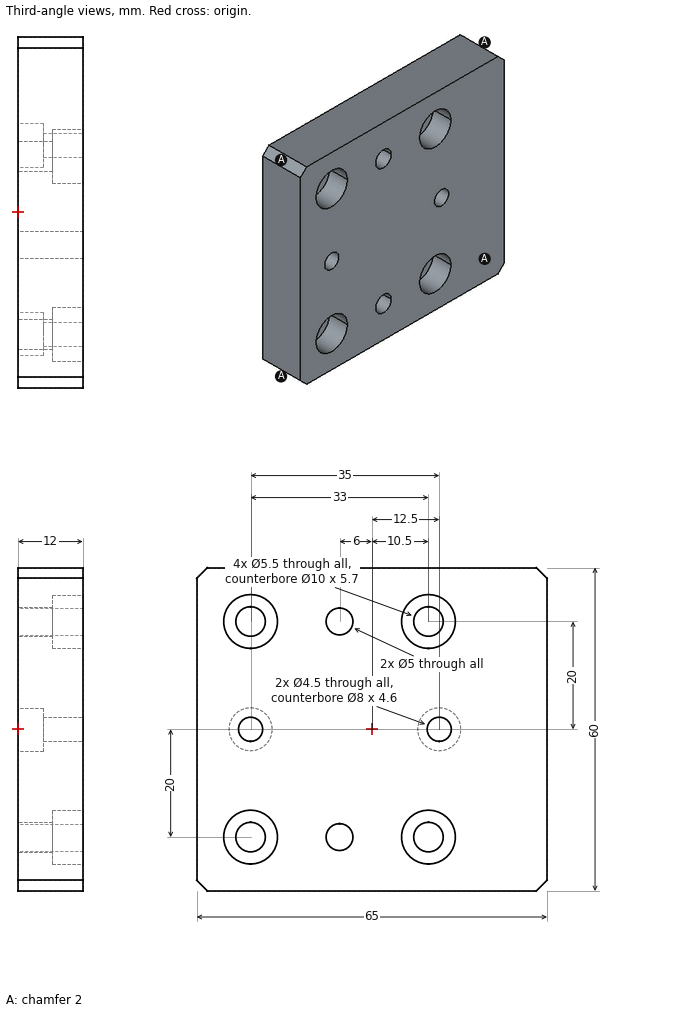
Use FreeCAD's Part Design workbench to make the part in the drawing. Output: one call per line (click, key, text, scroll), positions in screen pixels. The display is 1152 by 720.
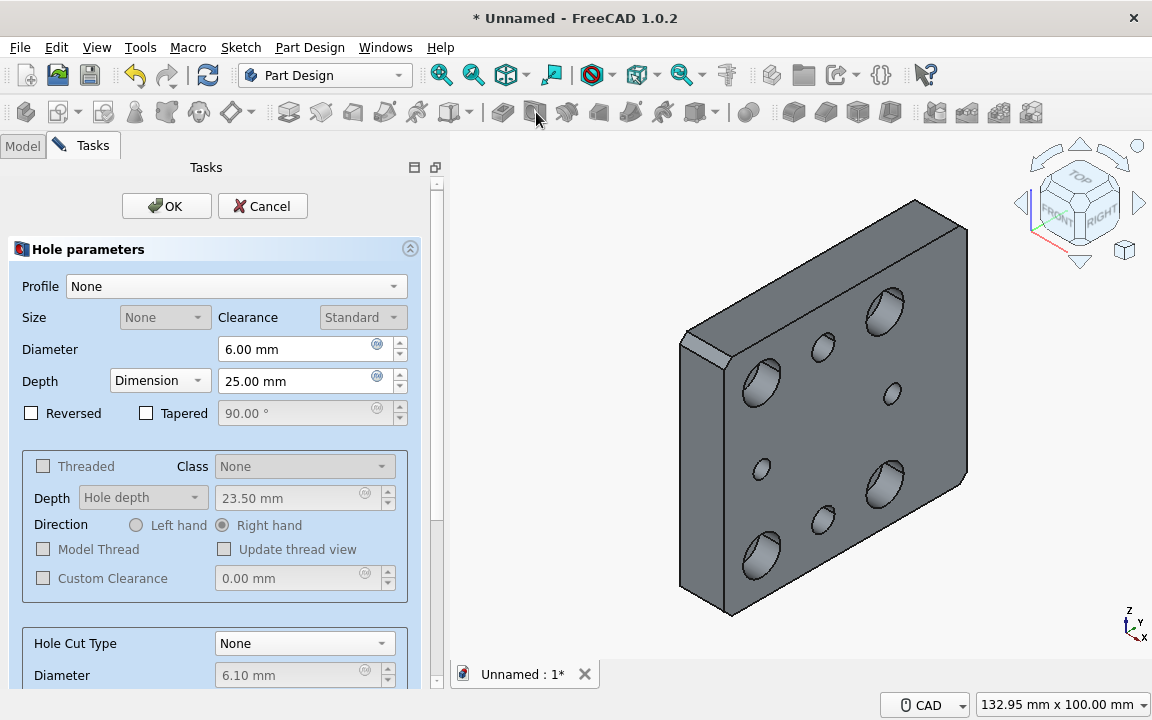
triple_click(305, 349)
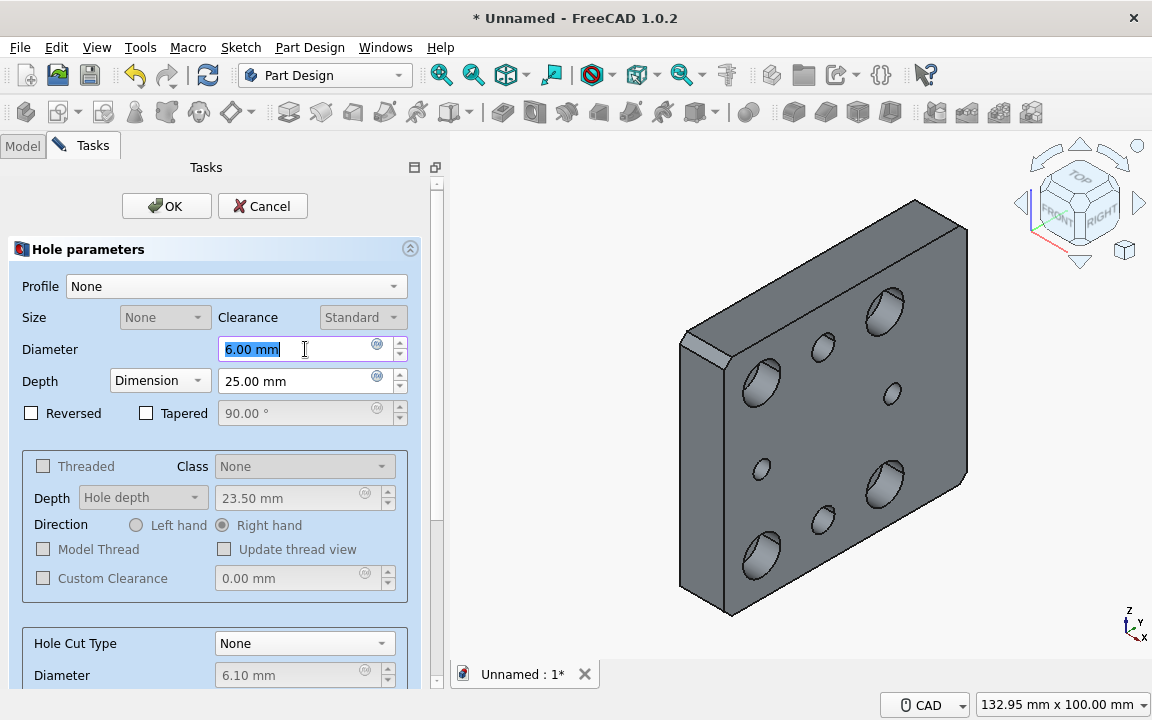
text(5)
key(Tab)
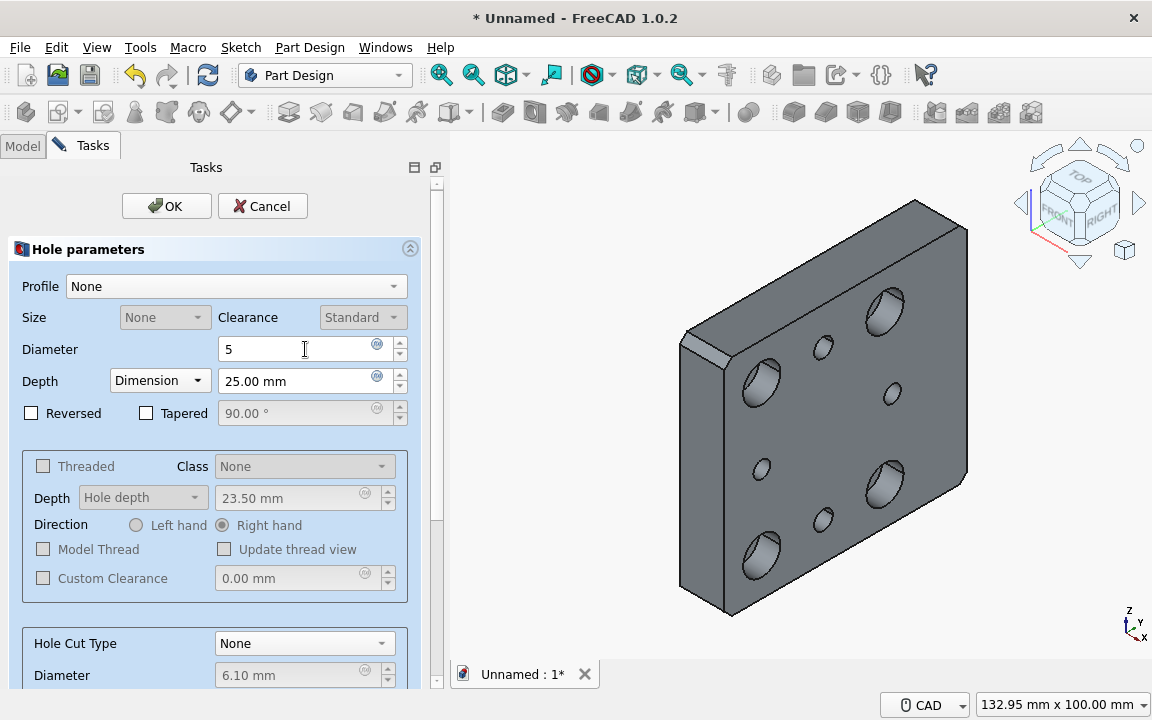
click(161, 380)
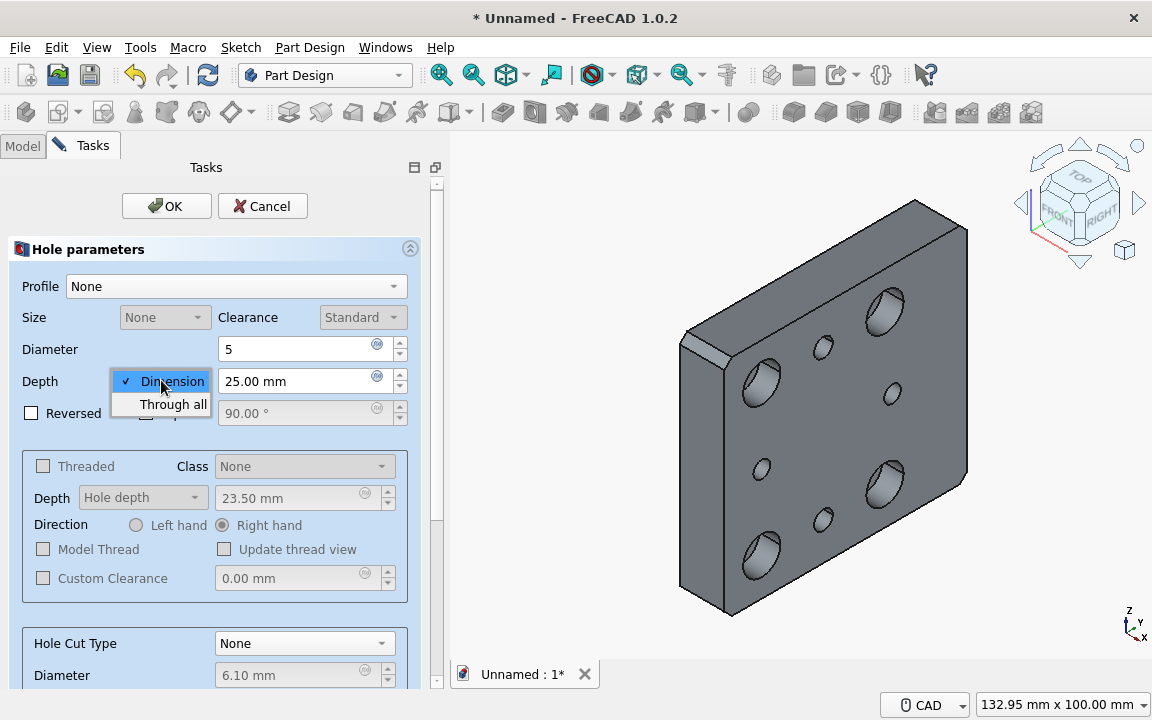
click(160, 404)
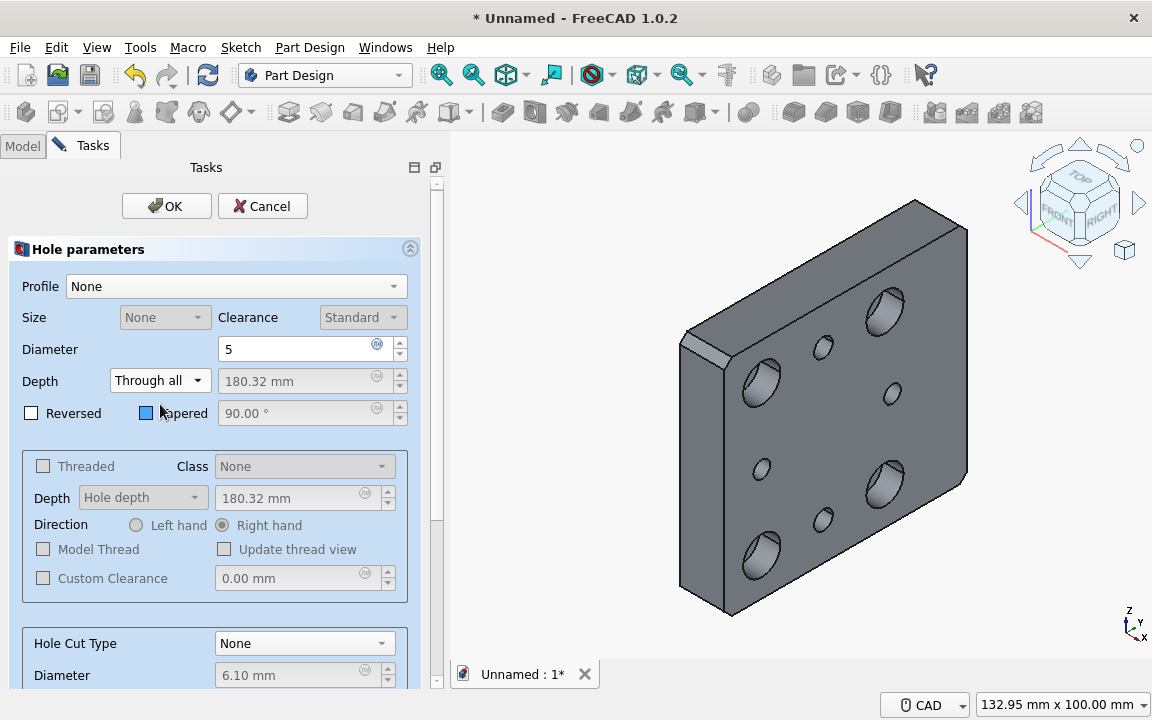
click(167, 206)